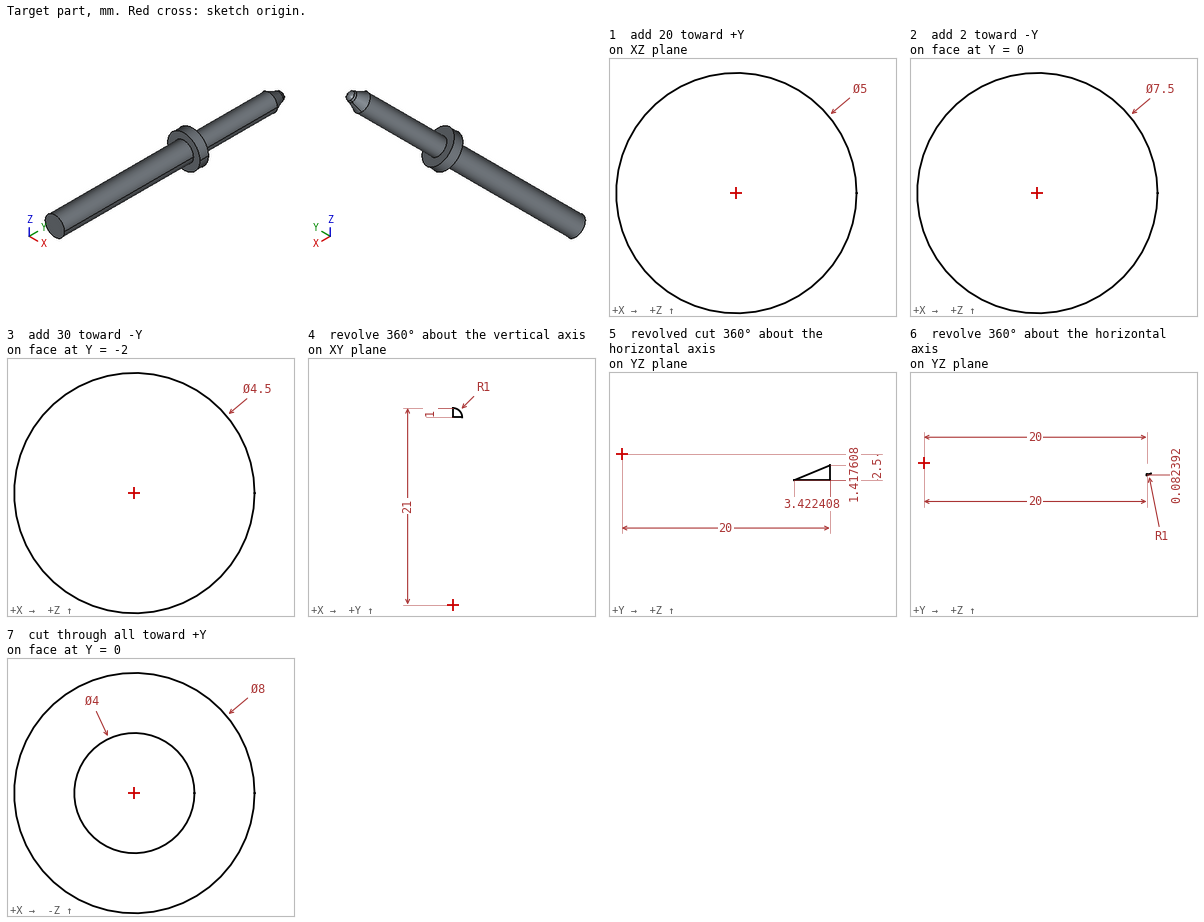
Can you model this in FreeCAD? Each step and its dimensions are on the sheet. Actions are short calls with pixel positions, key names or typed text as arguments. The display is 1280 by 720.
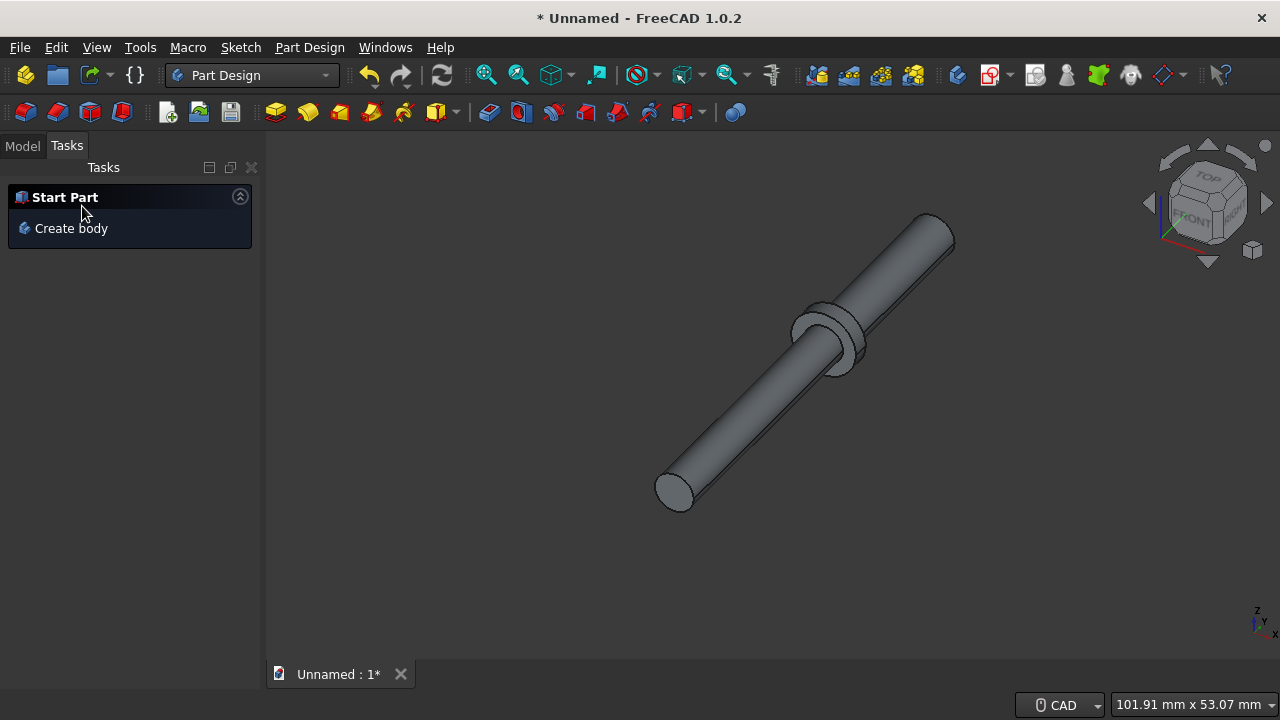
click(990, 76)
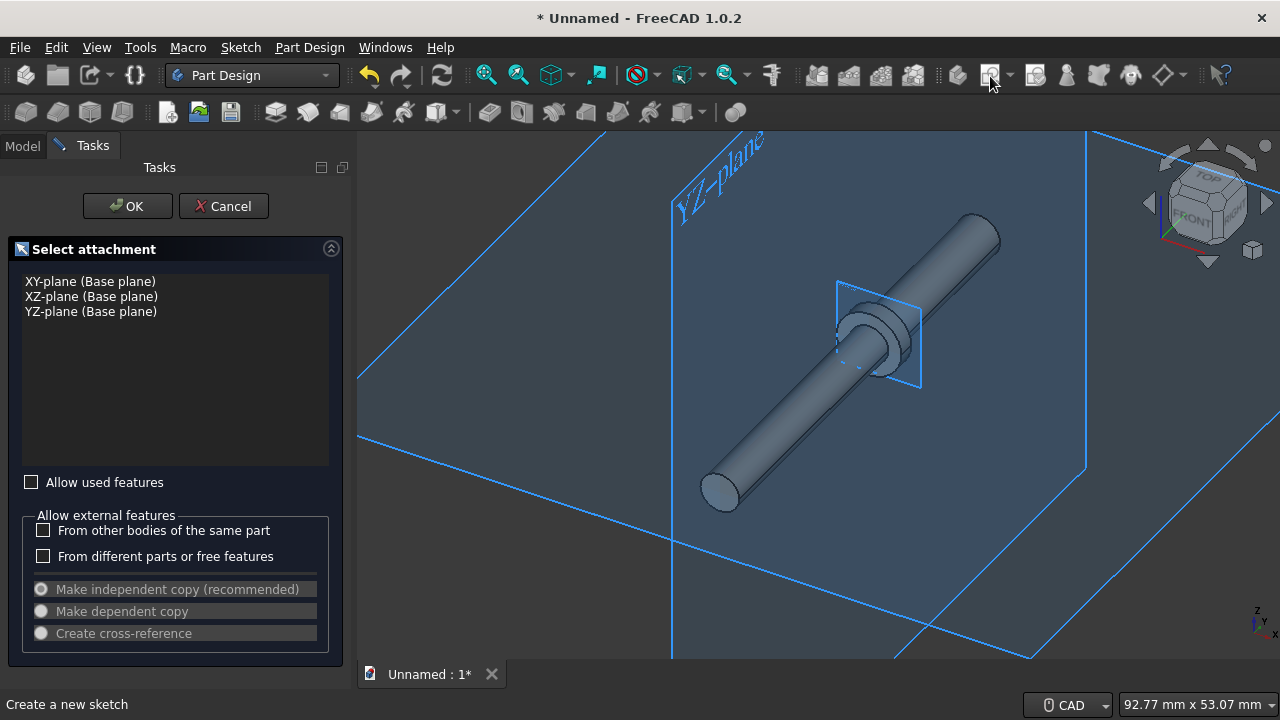
click(82, 312)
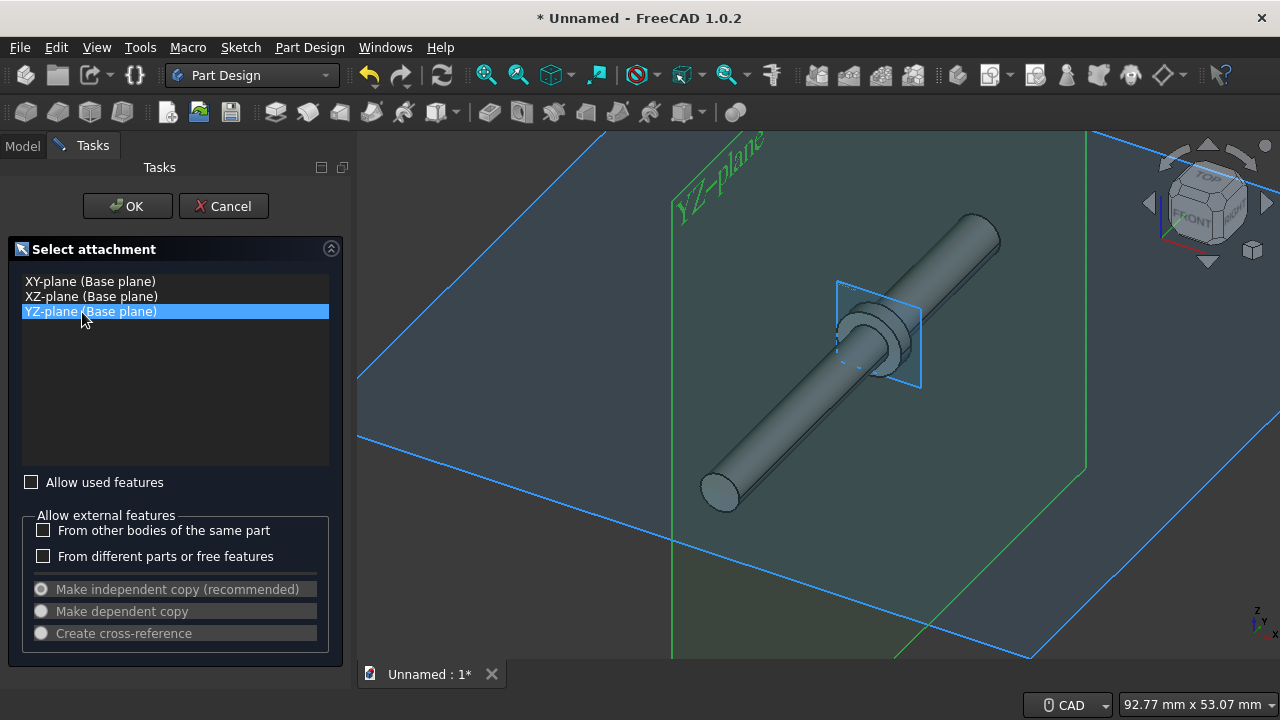
click(128, 206)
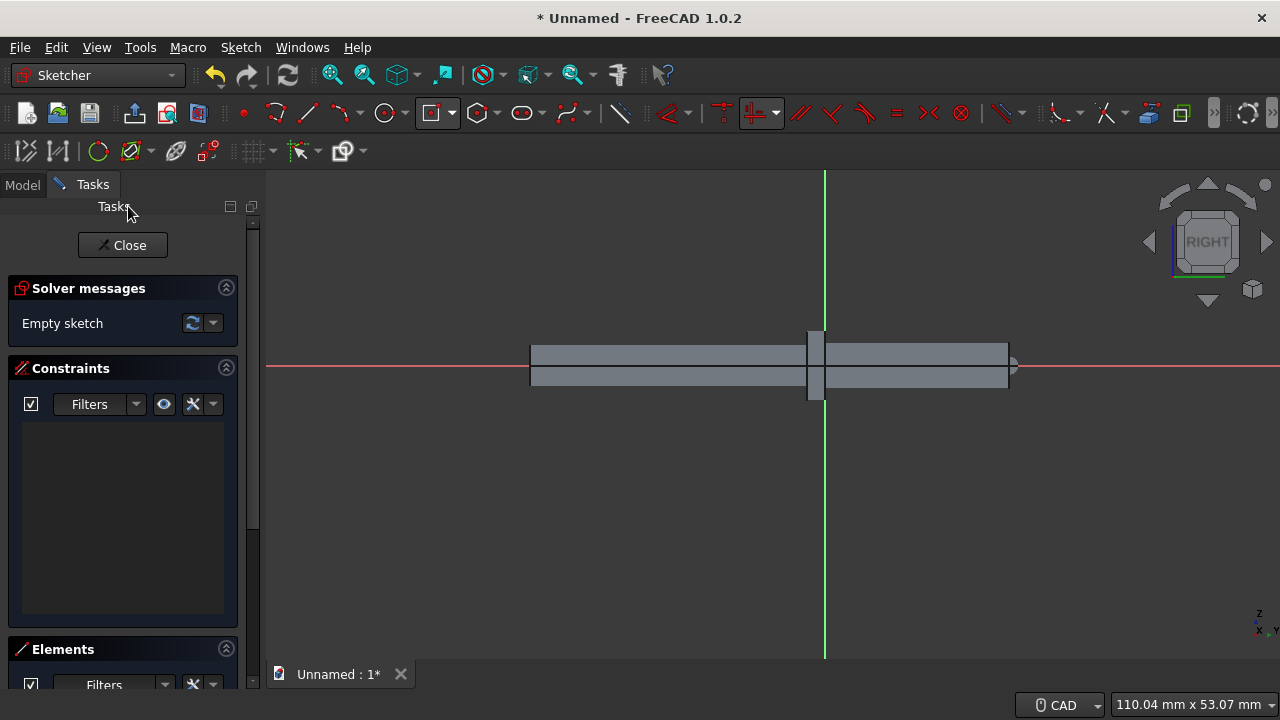
click(200, 114)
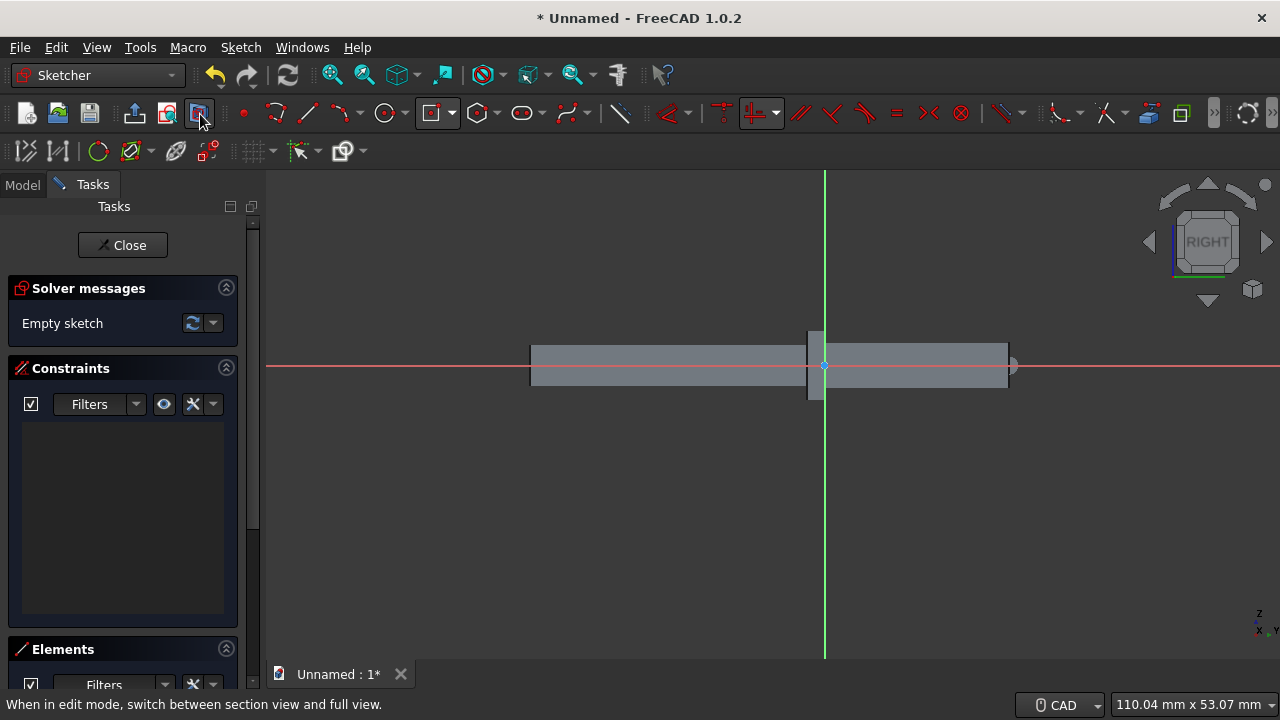
scroll(1009, 380, up, 15)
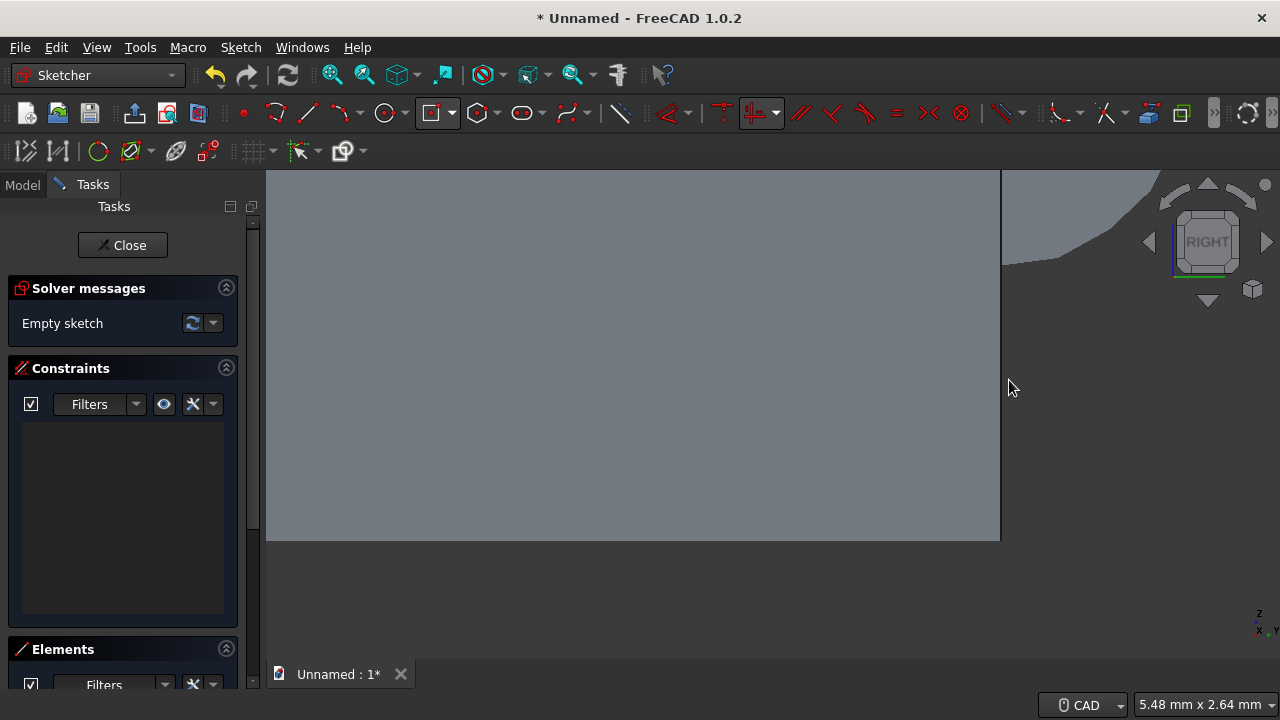
key(g)
key(m)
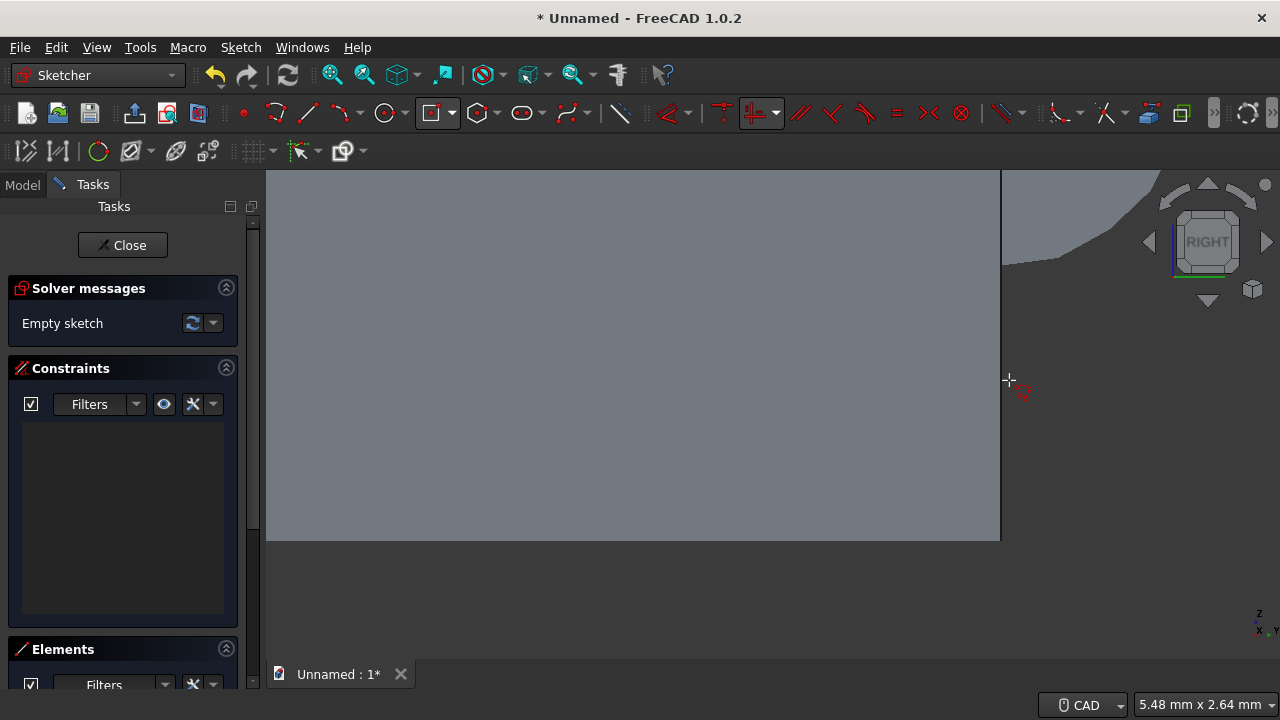
click(367, 545)
click(1001, 545)
click(1001, 282)
click(367, 546)
key(Escape)
key(Escape)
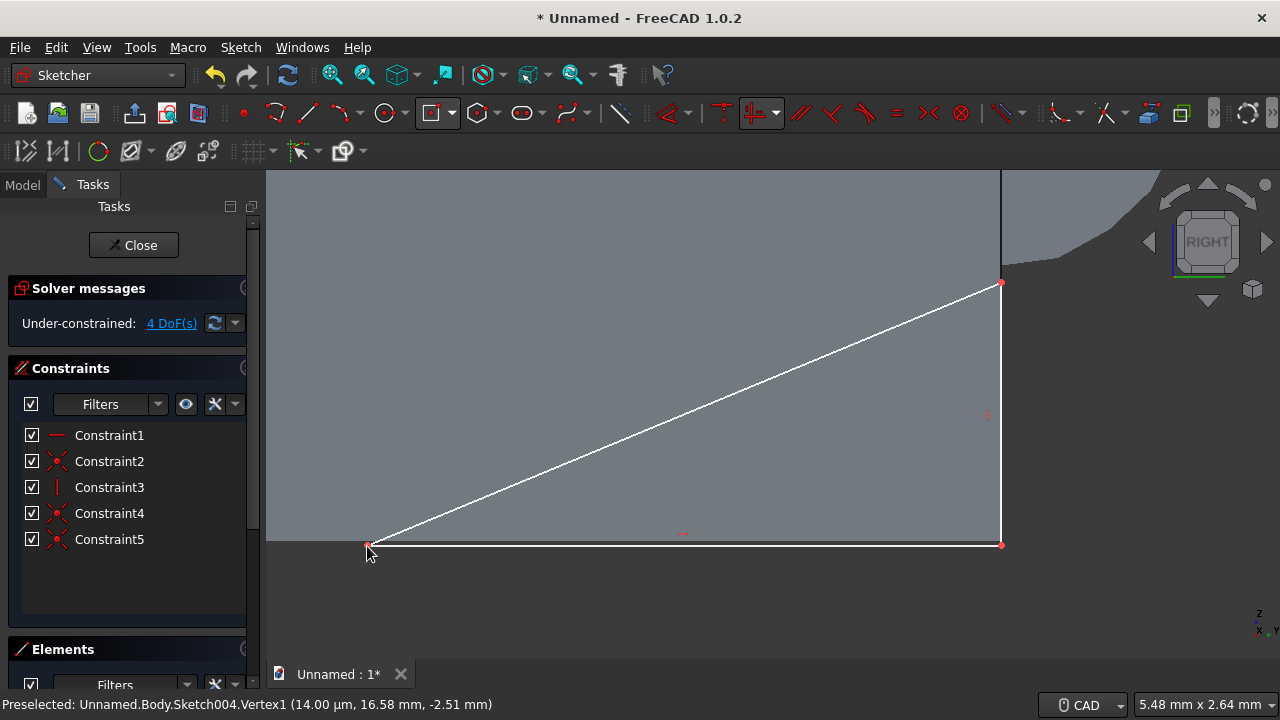
click(668, 114)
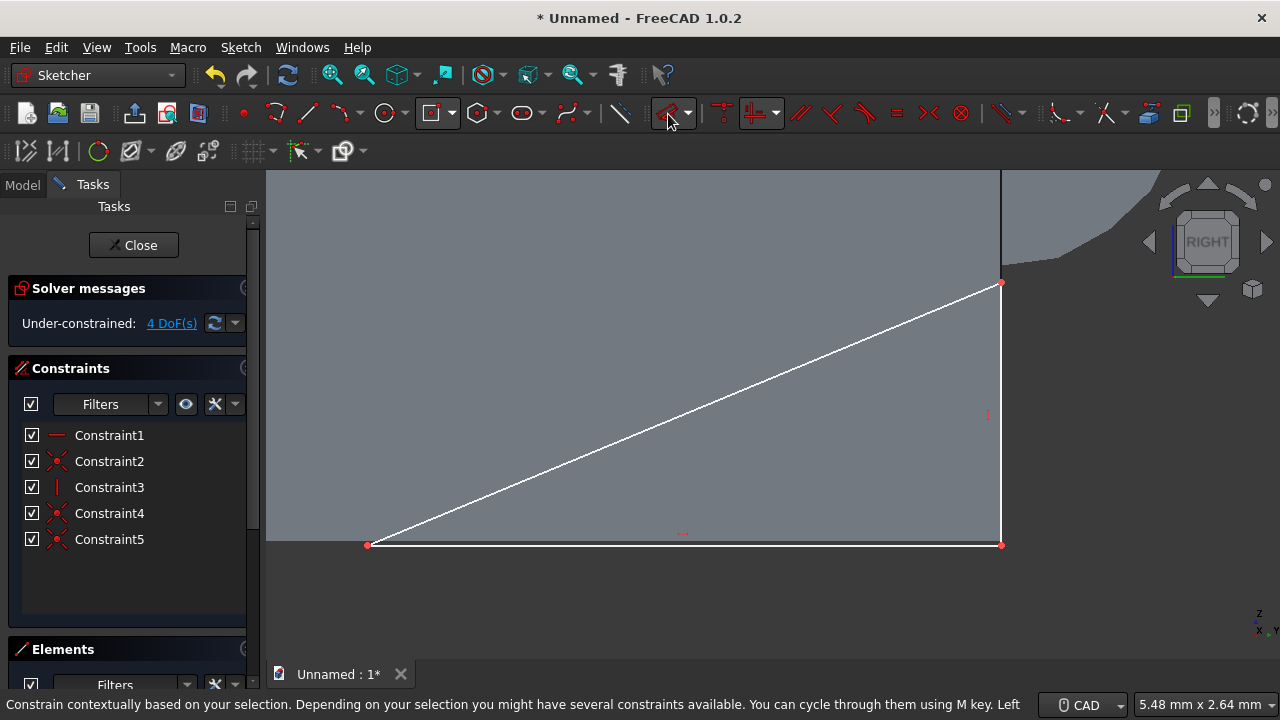
click(1001, 546)
click(648, 580)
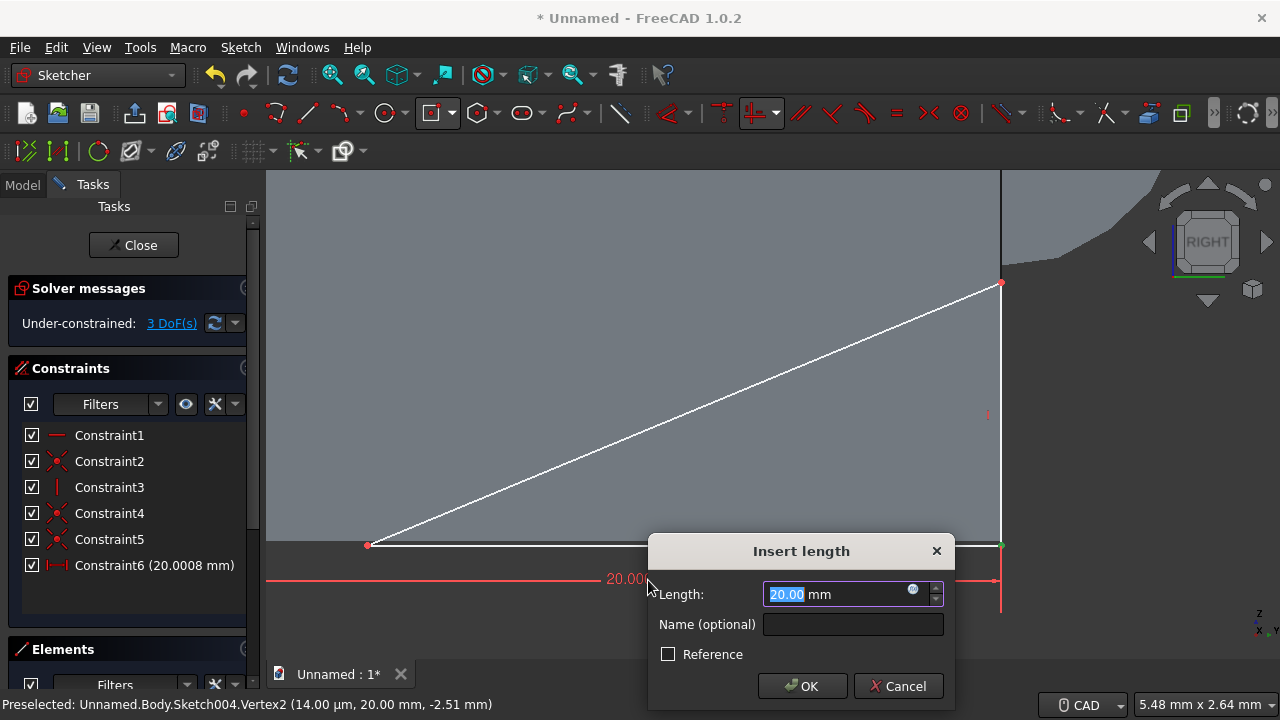
text(20)
key(Return)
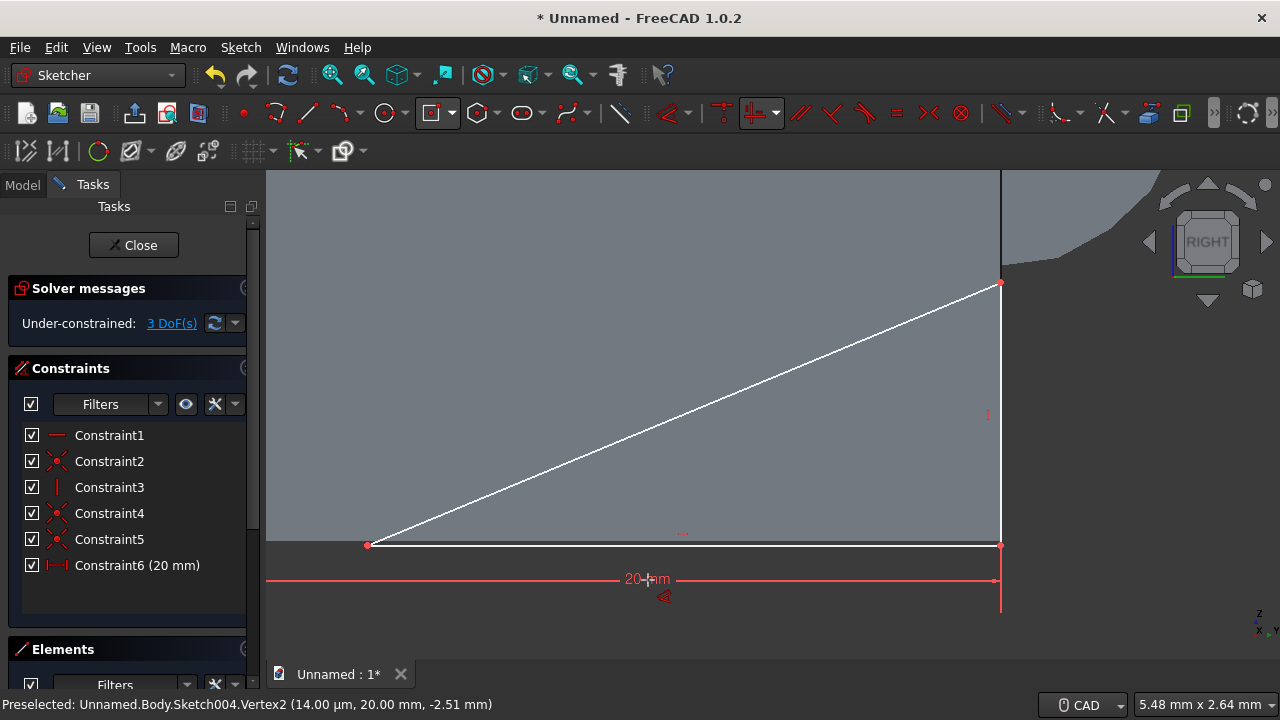
click(367, 546)
click(401, 372)